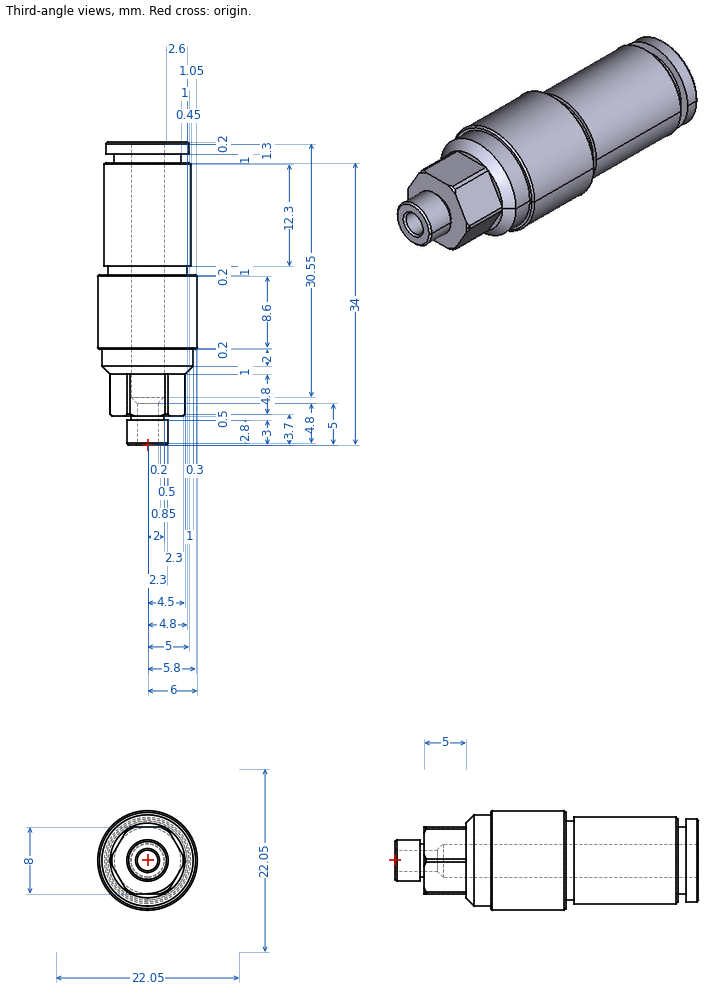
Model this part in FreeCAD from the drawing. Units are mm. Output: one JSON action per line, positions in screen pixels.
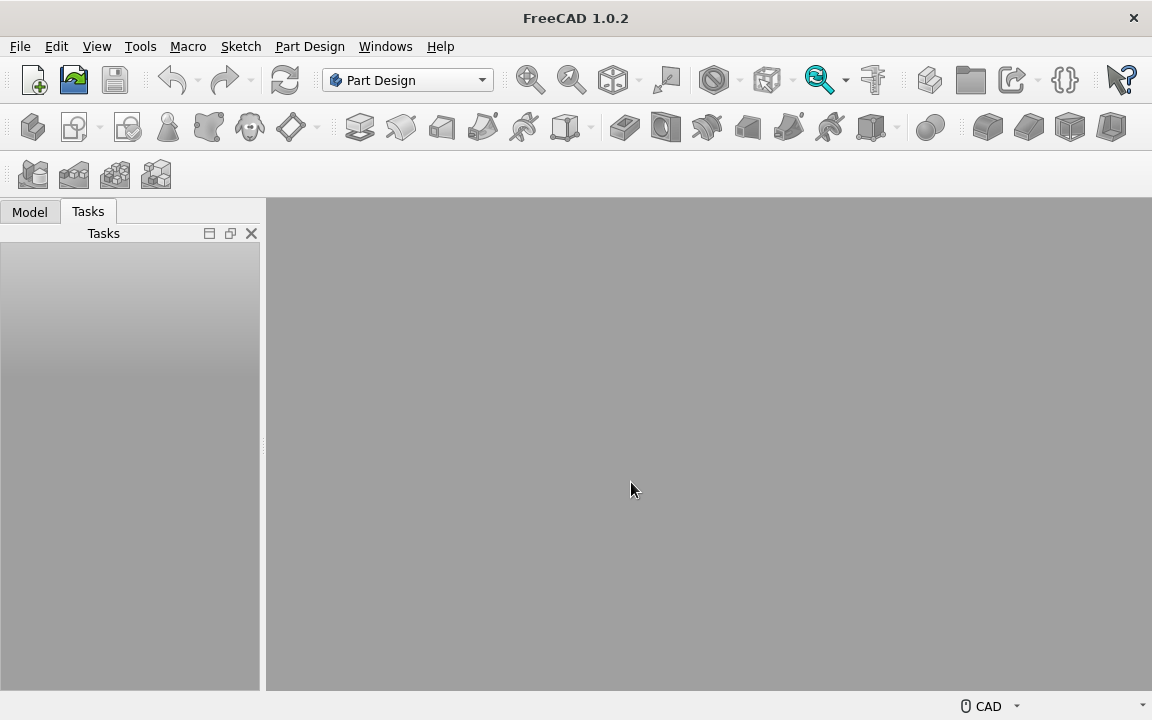
{"action": "key", "text": "ctrl+n"}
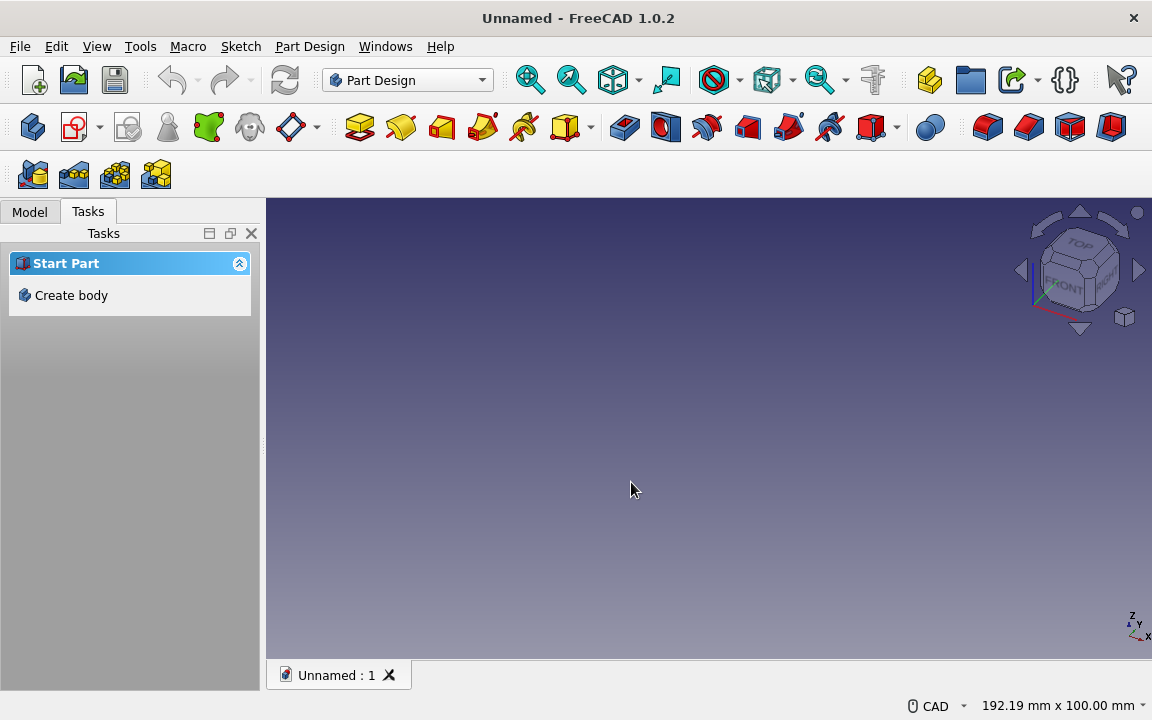
{"action": "left_click", "coordinate": [74, 128]}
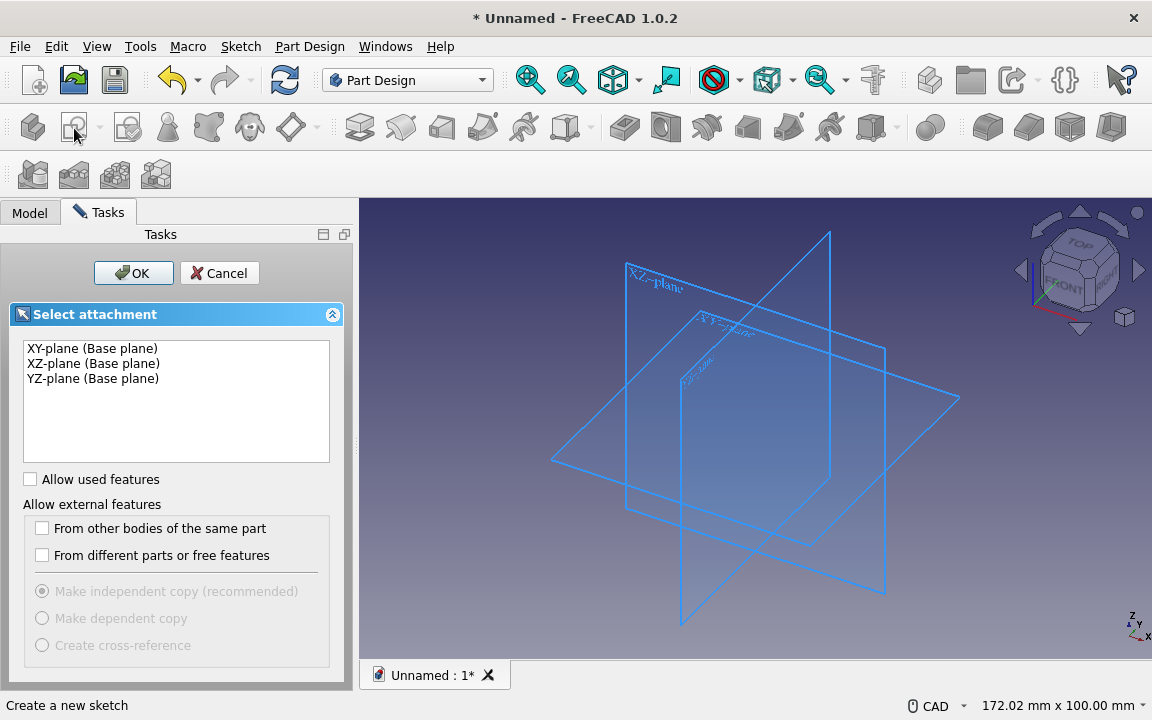
{"action": "left_click", "coordinate": [84, 348]}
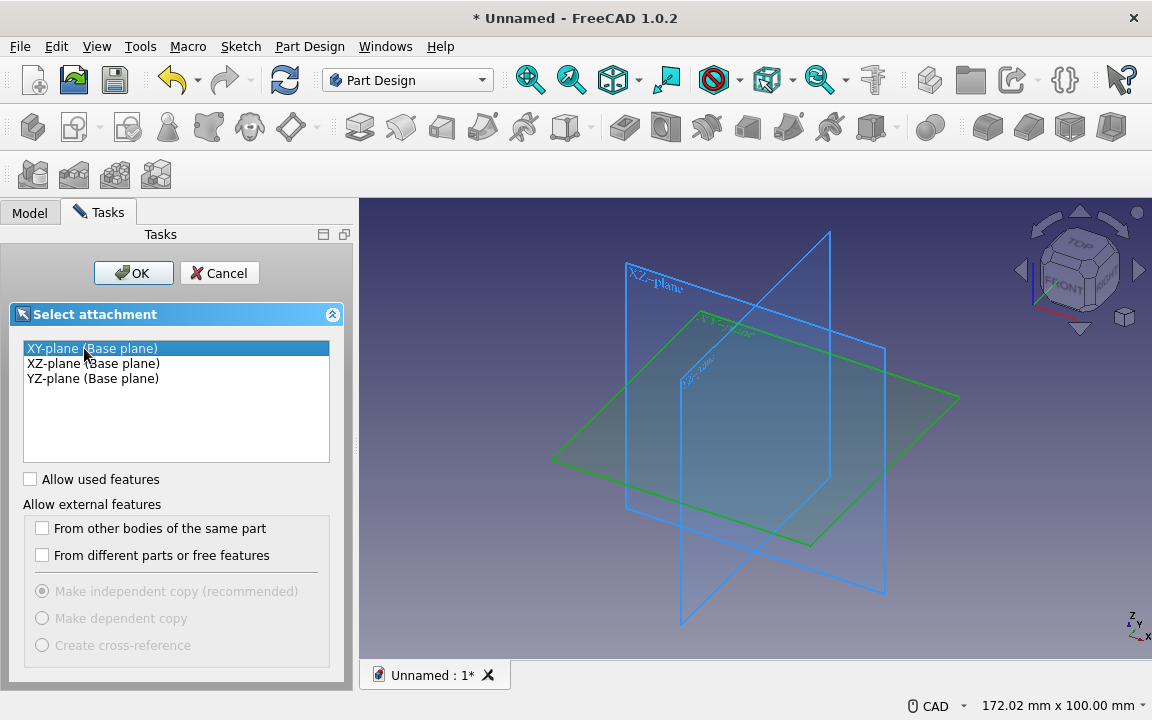
{"action": "left_click", "coordinate": [134, 273]}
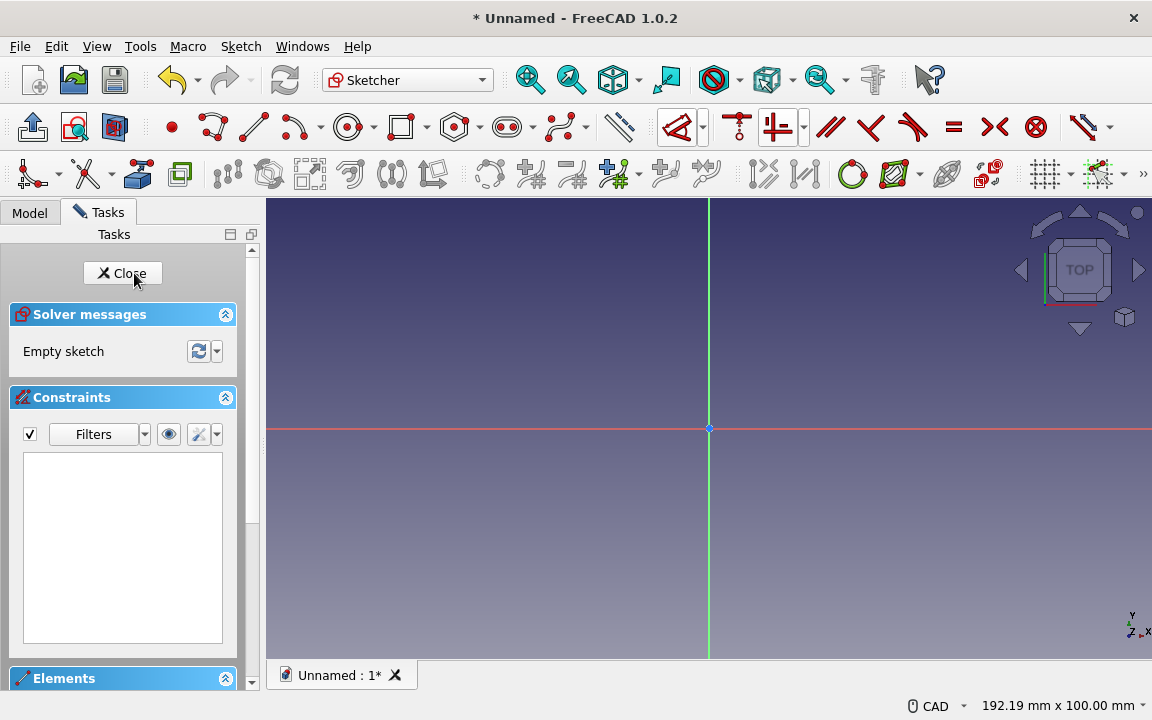
{"action": "scroll", "coordinate": [823, 242], "scroll_direction": "up", "scroll_amount": 3}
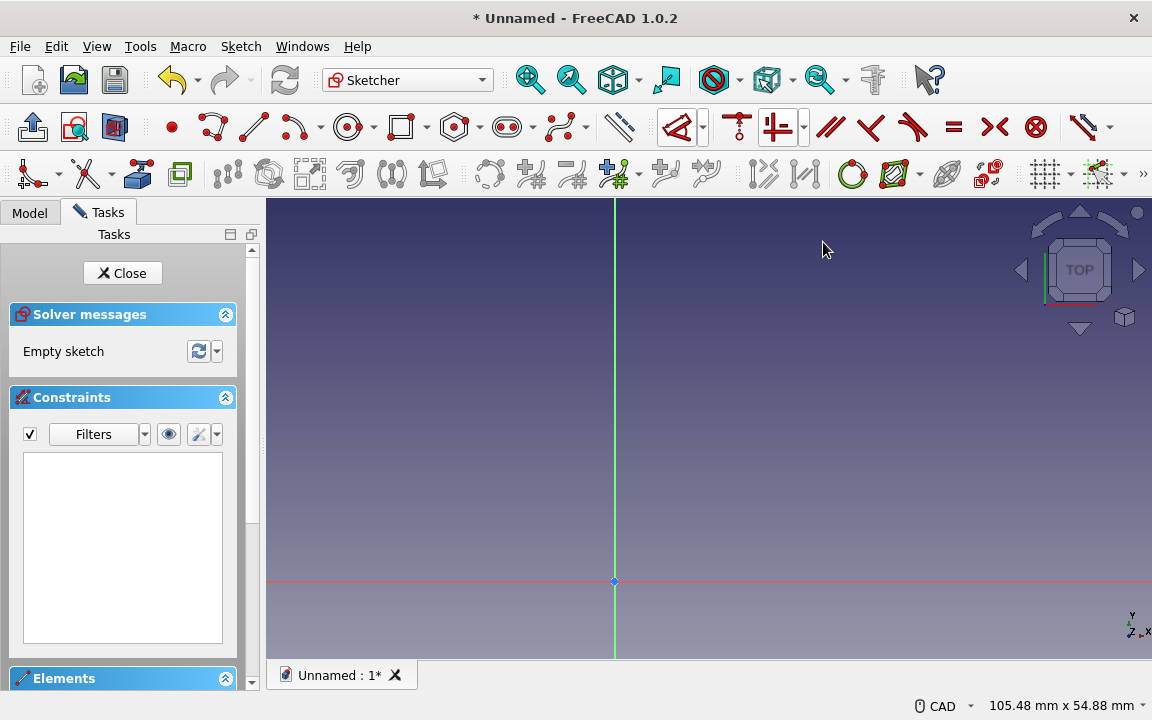
{"action": "left_click", "coordinate": [213, 128]}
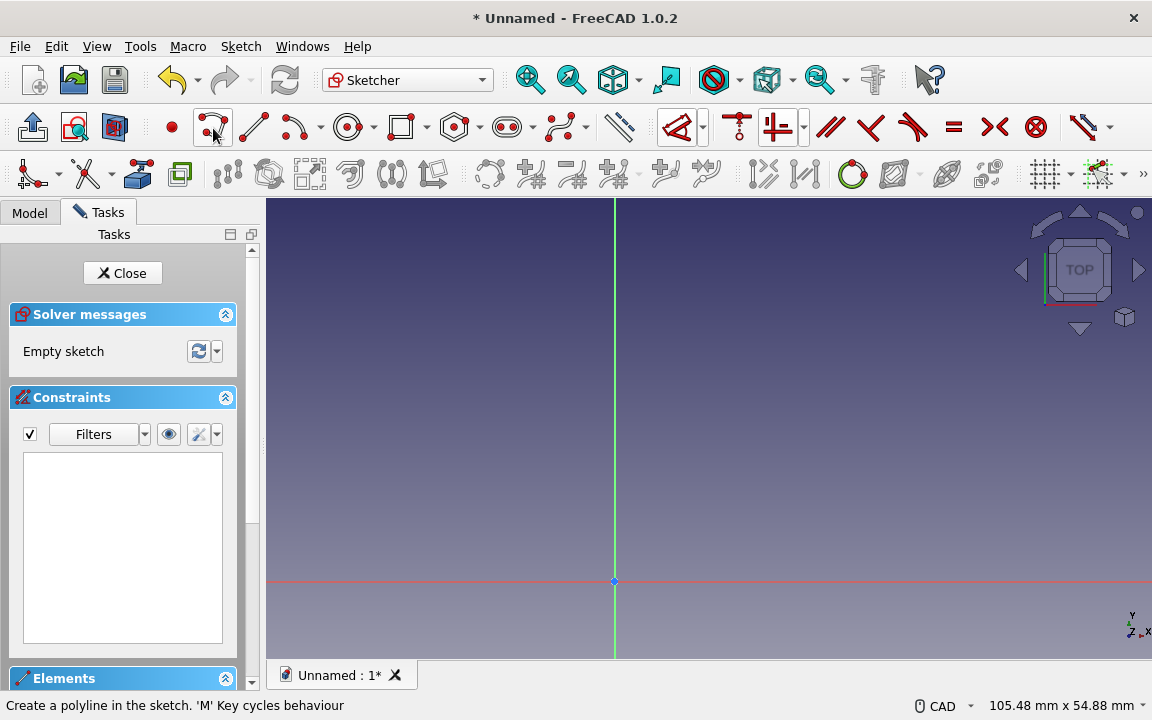
{"action": "scroll", "coordinate": [625, 580], "scroll_direction": "up", "scroll_amount": 12}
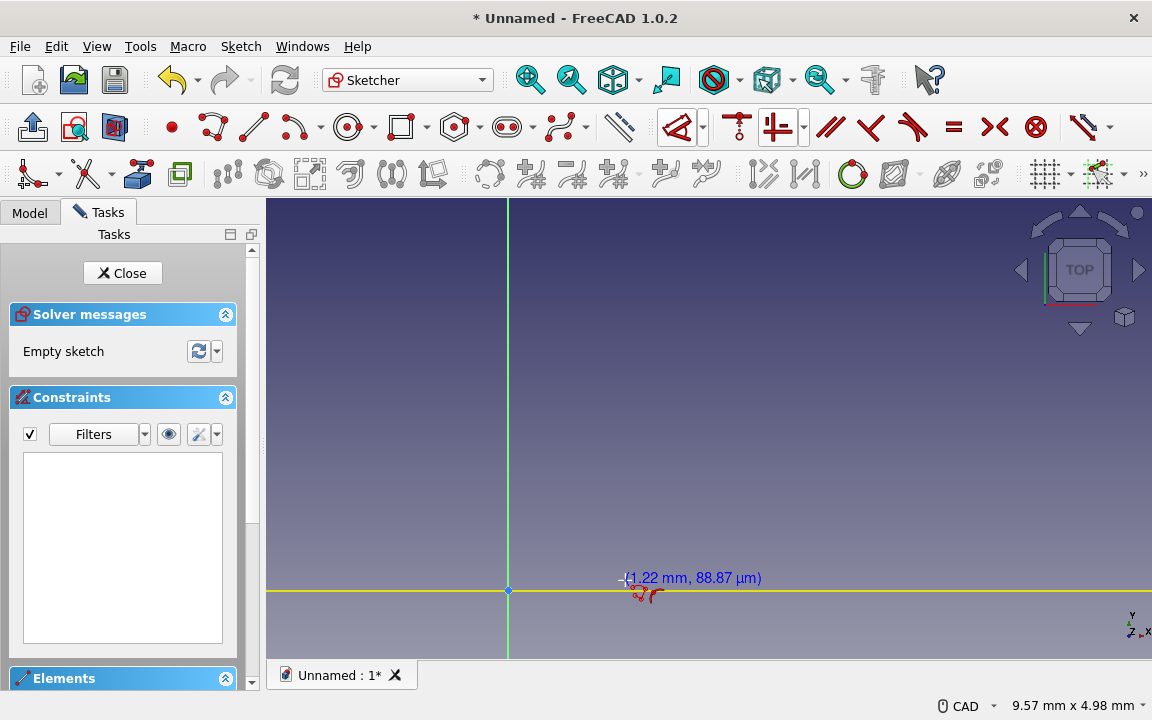
{"action": "left_click", "coordinate": [624, 572]}
{"action": "left_click", "coordinate": [642, 591]}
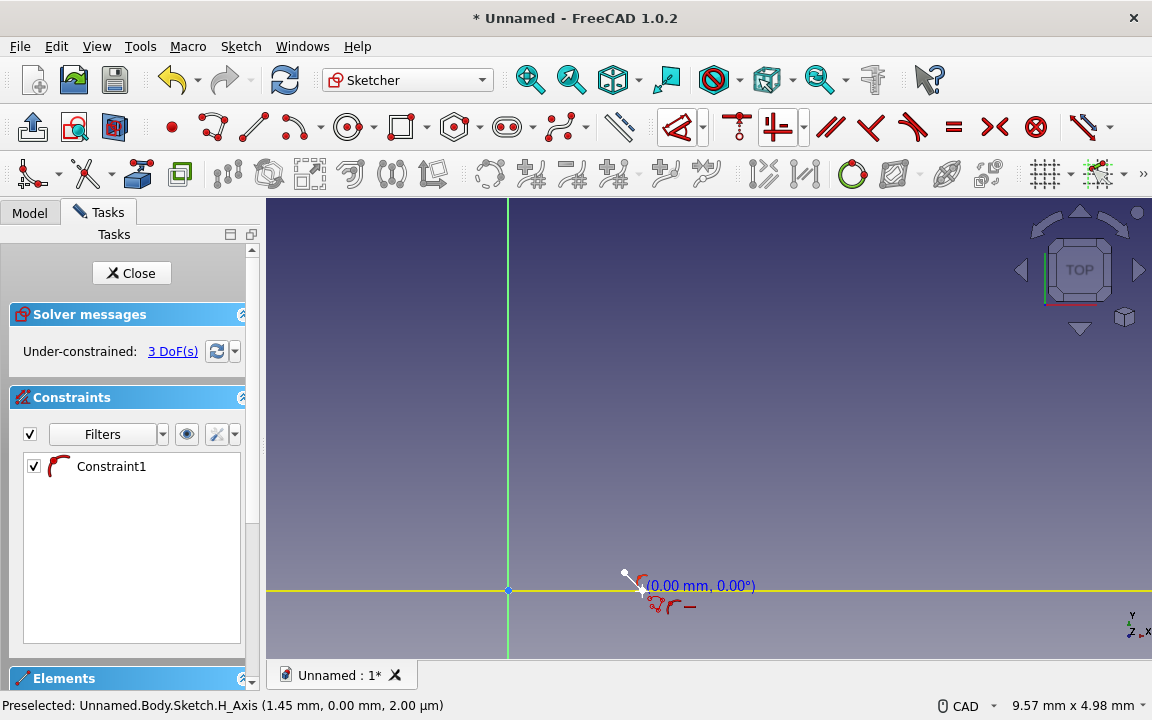
{"action": "scroll", "coordinate": [626, 581], "scroll_direction": "down", "scroll_amount": 12}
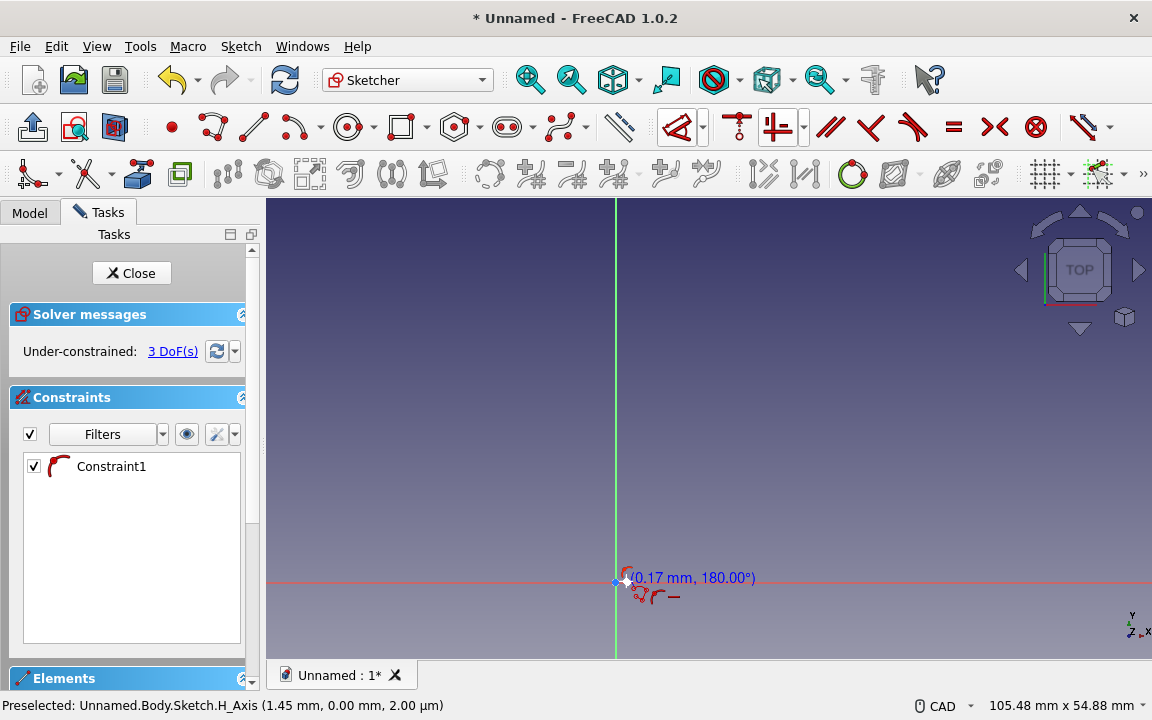
{"action": "scroll", "coordinate": [635, 583], "scroll_direction": "up", "scroll_amount": 4}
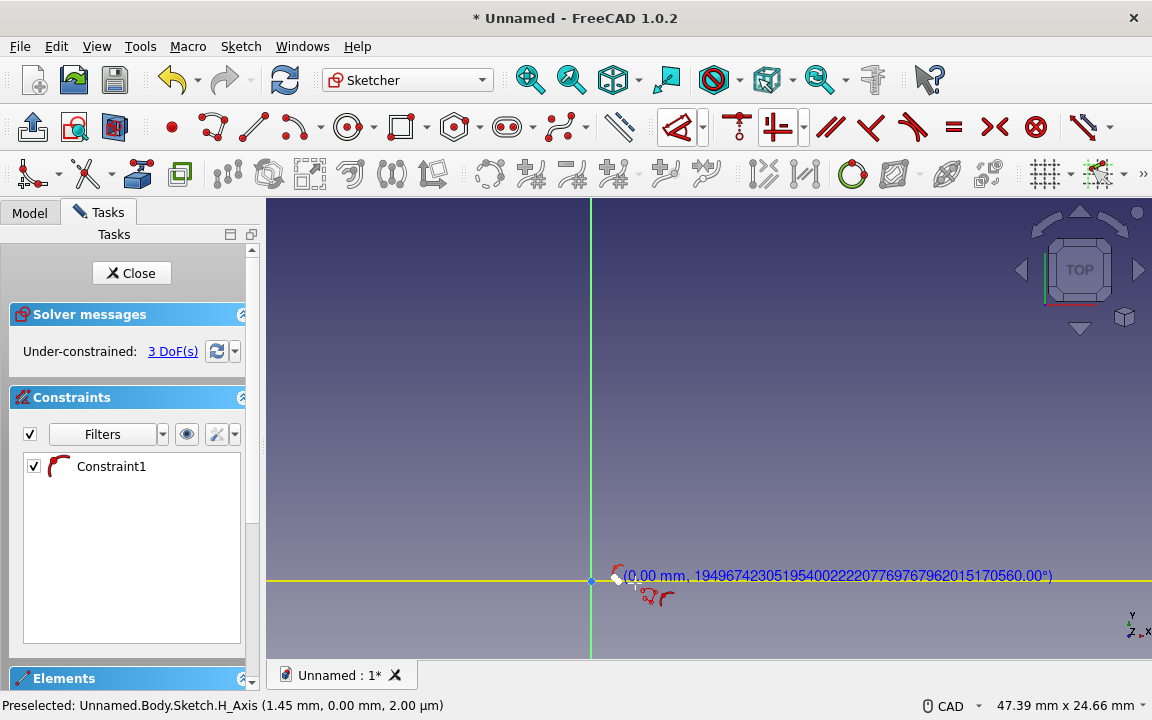
{"action": "left_click", "coordinate": [634, 572]}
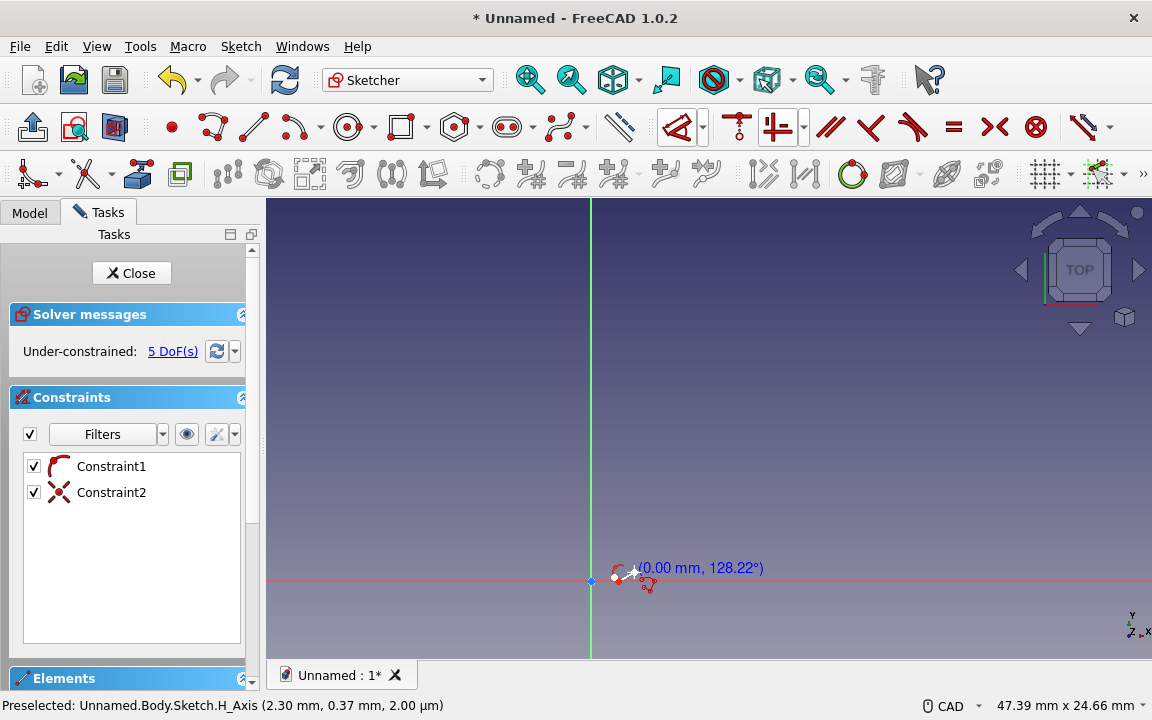
{"action": "scroll", "coordinate": [638, 577], "scroll_direction": "up", "scroll_amount": 8}